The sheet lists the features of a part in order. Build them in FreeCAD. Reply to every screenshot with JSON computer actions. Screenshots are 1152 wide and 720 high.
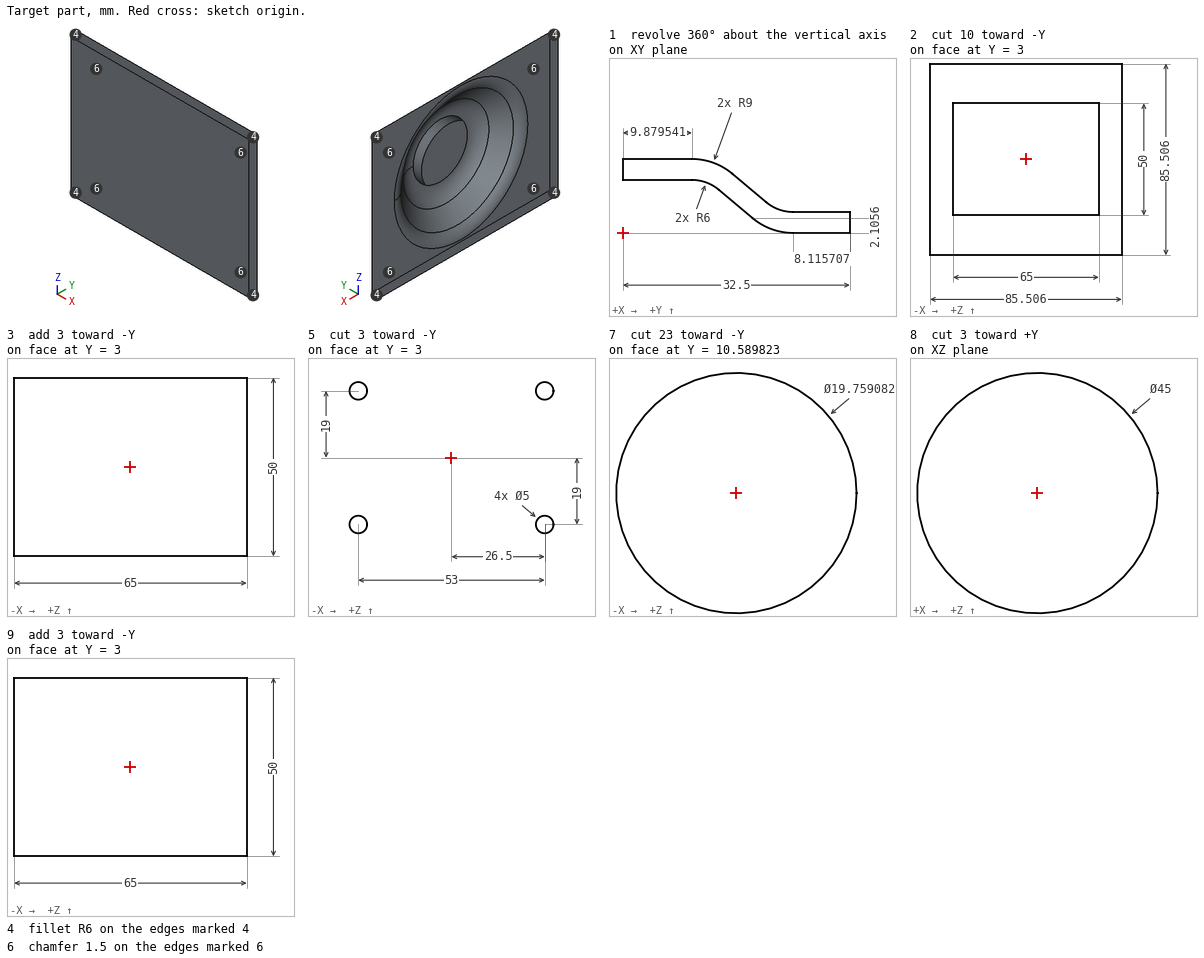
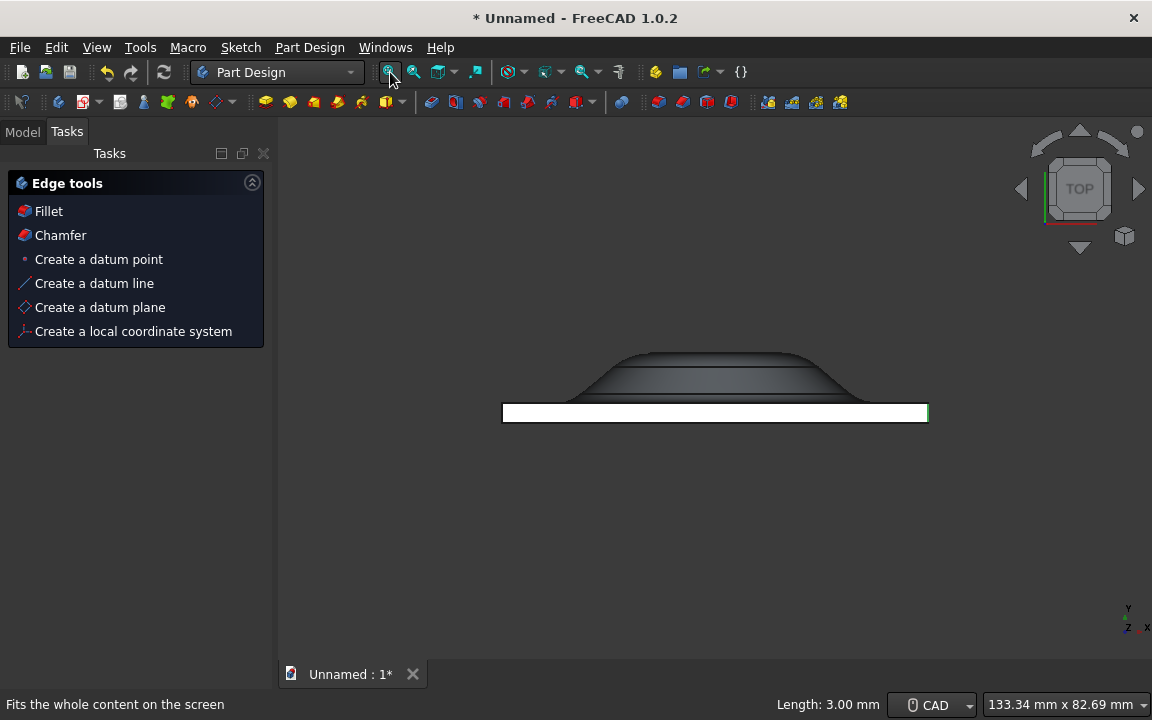
{"action": "left_click", "coordinate": [502, 412], "text": "ctrl"}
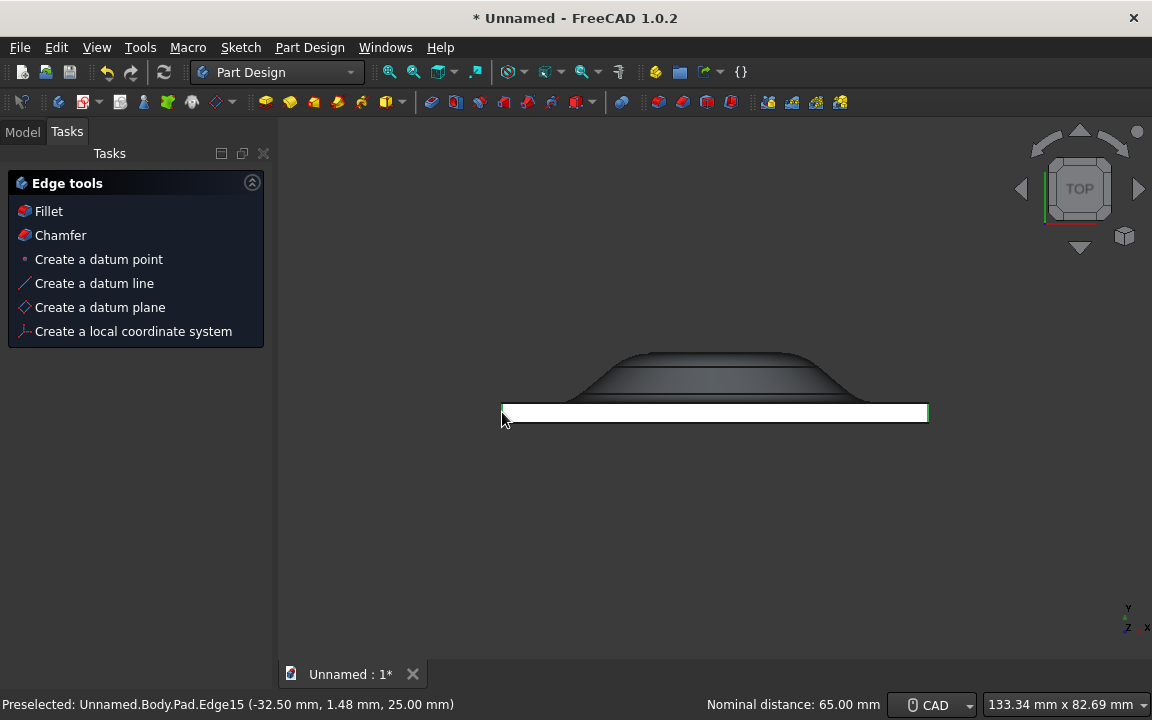
{"action": "scroll", "coordinate": [928, 412], "scroll_direction": "up", "scroll_amount": 4}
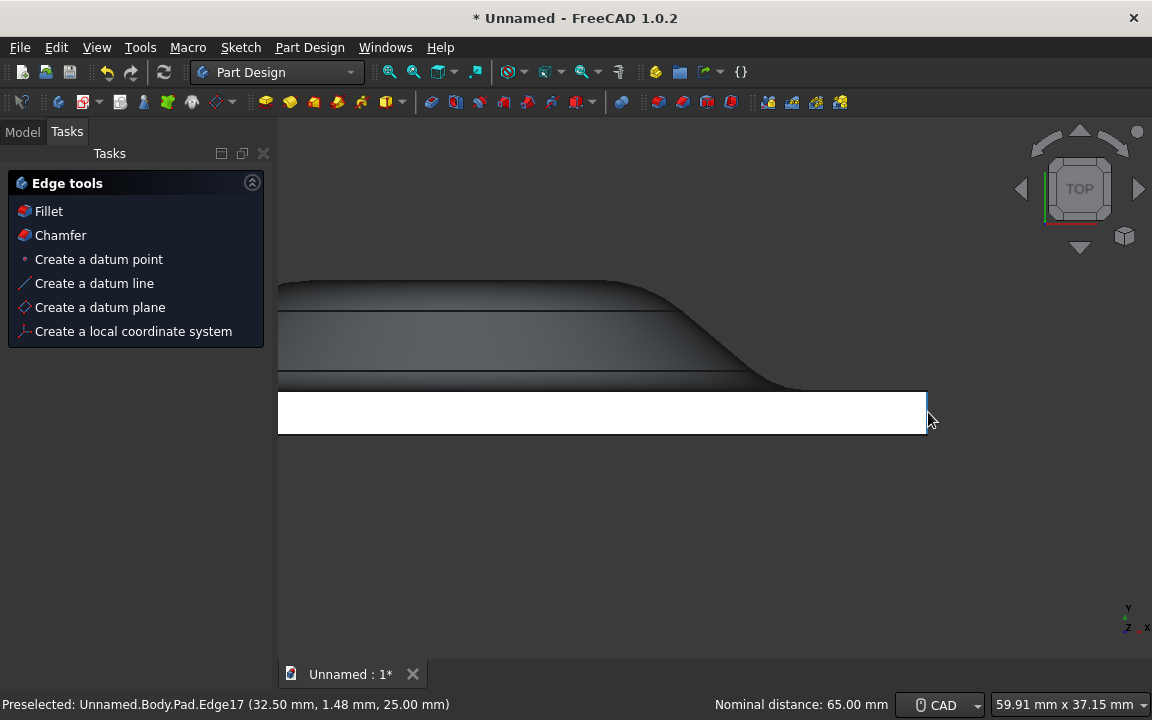
{"action": "left_click", "coordinate": [390, 72]}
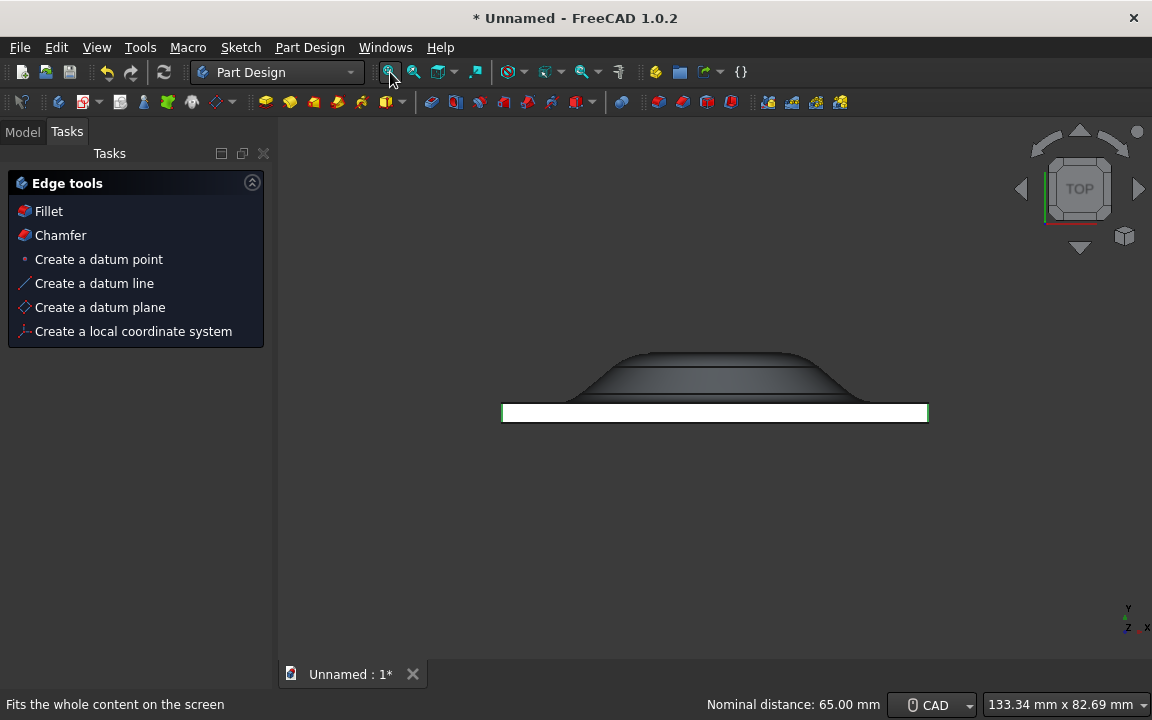
{"action": "key", "text": "1"}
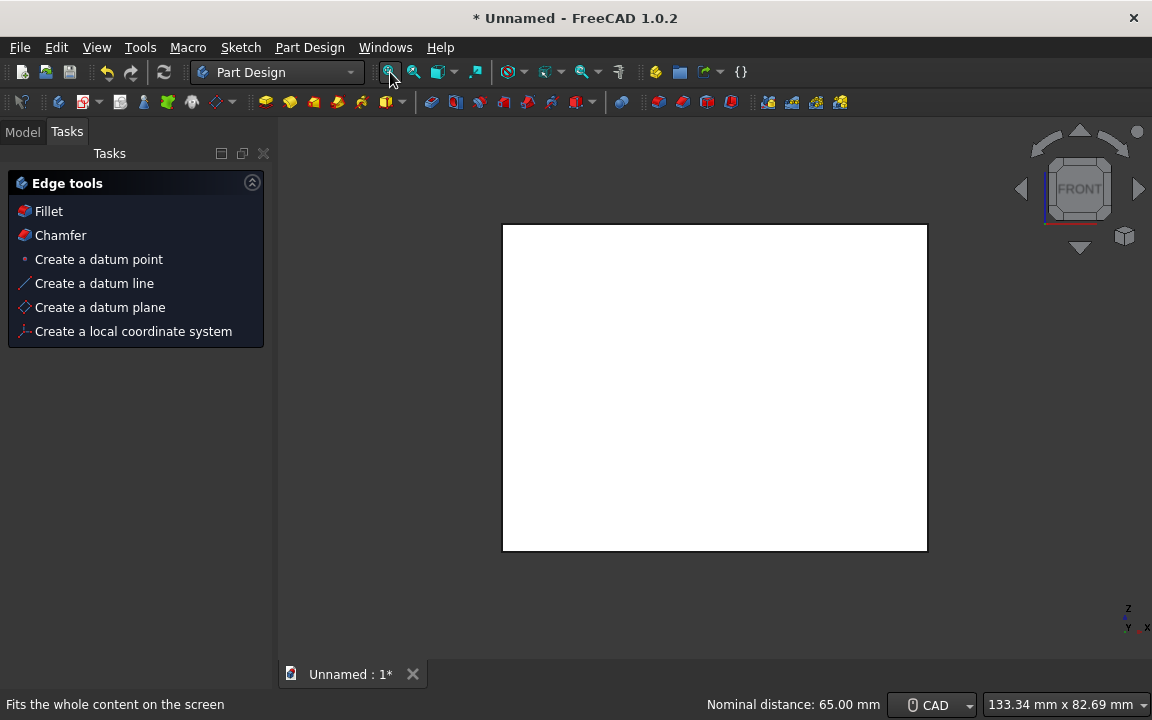
{"action": "scroll", "coordinate": [928, 551], "scroll_direction": "up", "scroll_amount": 4}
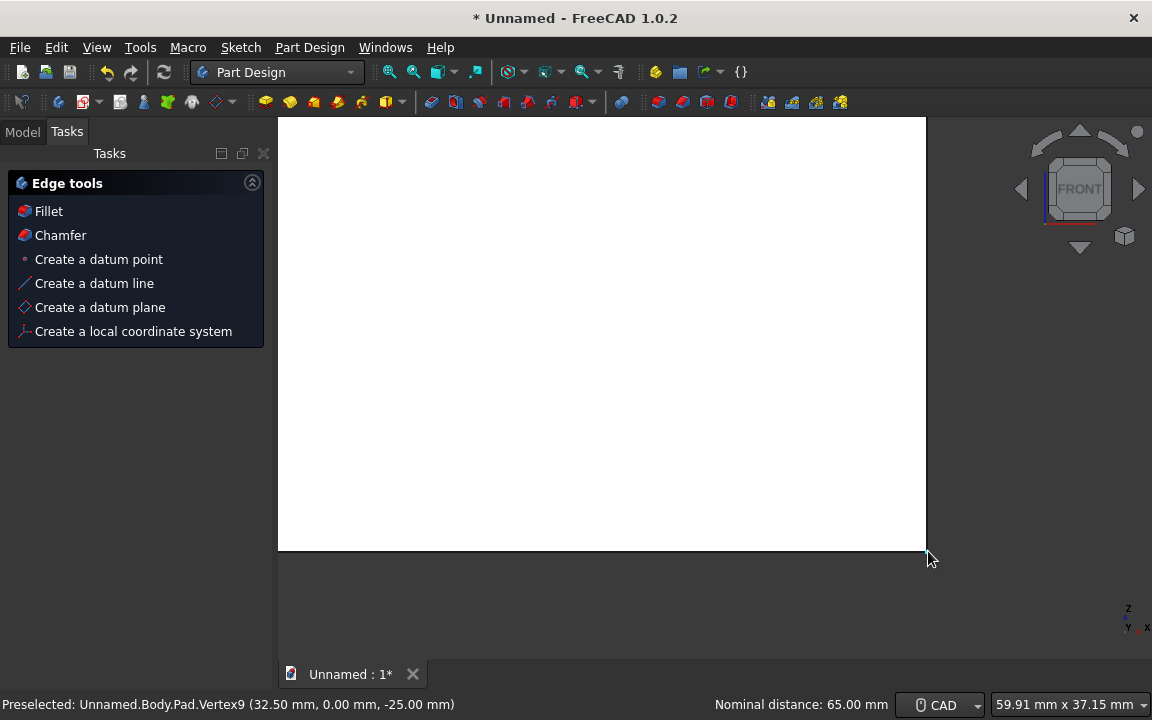
{"action": "left_click", "coordinate": [390, 72]}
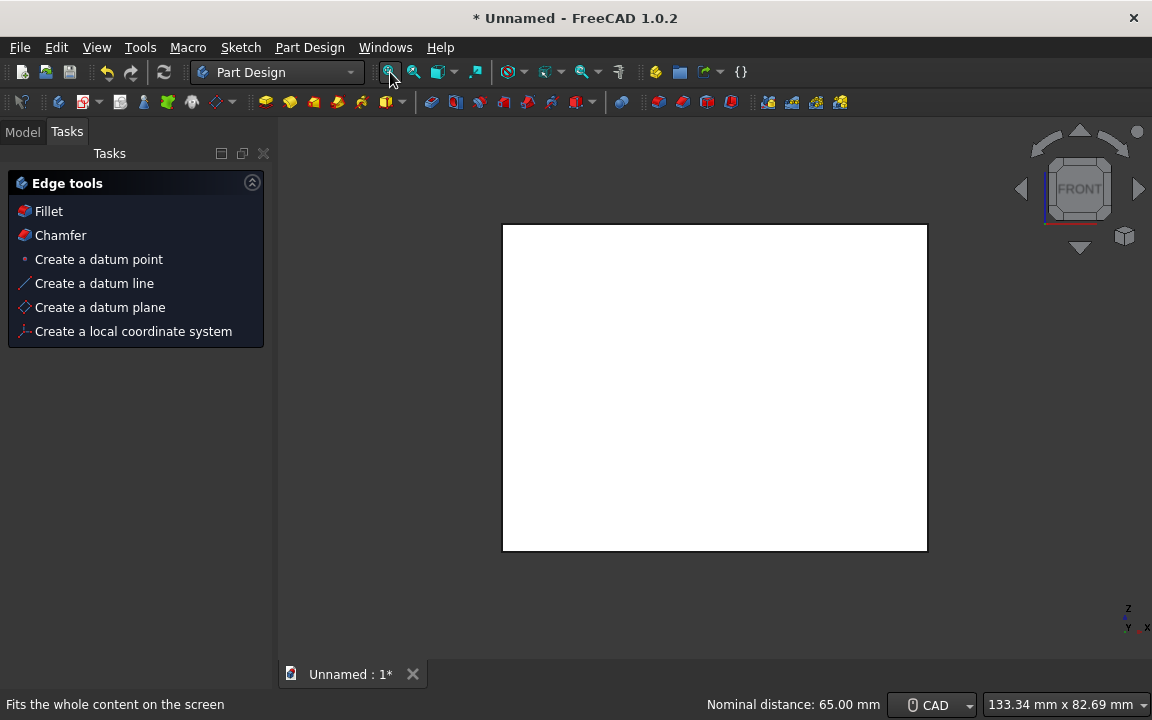
{"action": "key", "text": "3"}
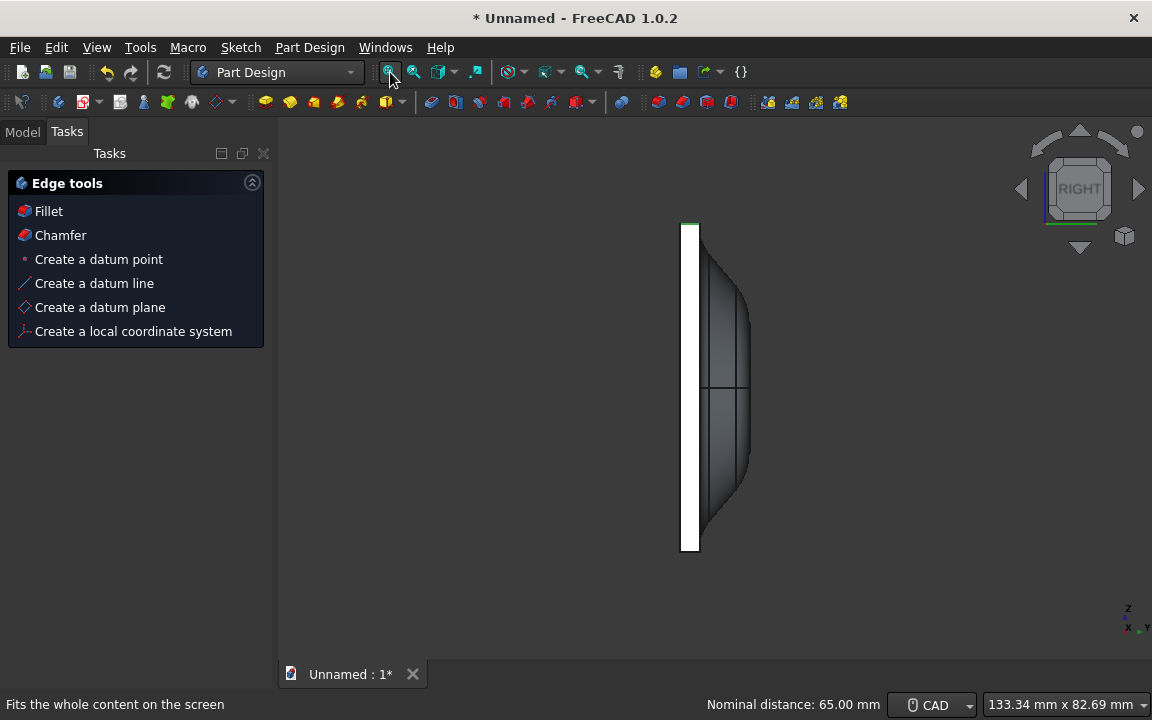
{"action": "left_click", "coordinate": [690, 551], "text": "ctrl"}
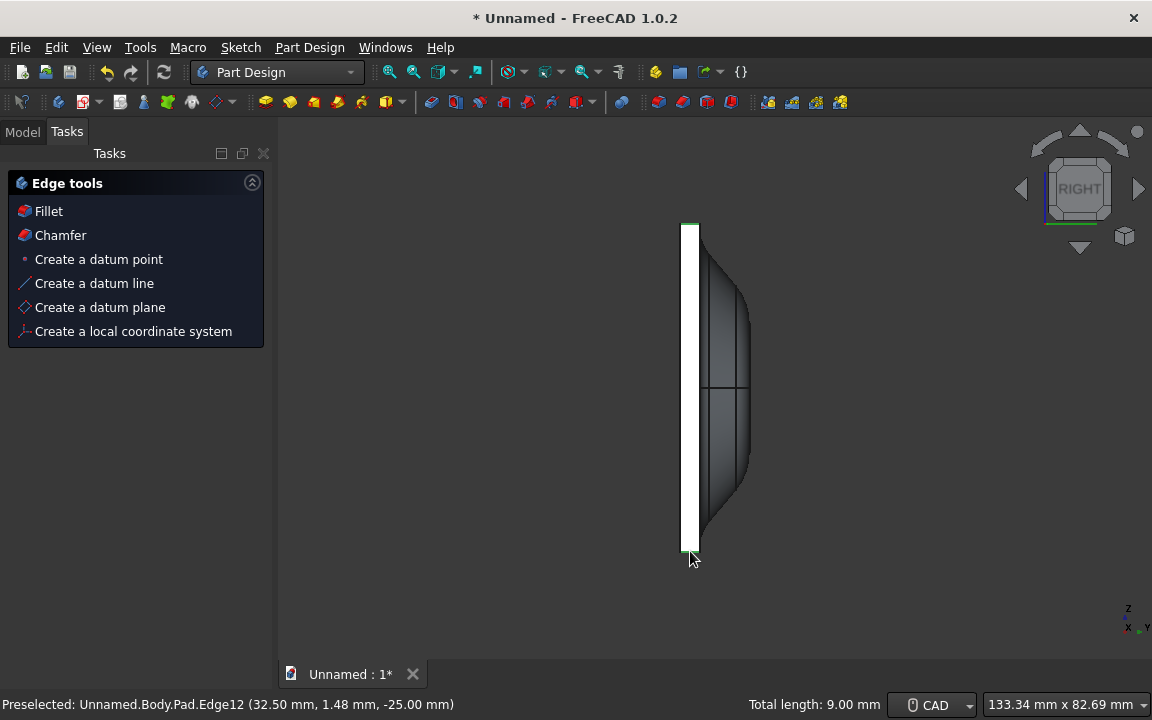
{"action": "scroll", "coordinate": [690, 551], "scroll_direction": "up", "scroll_amount": 4}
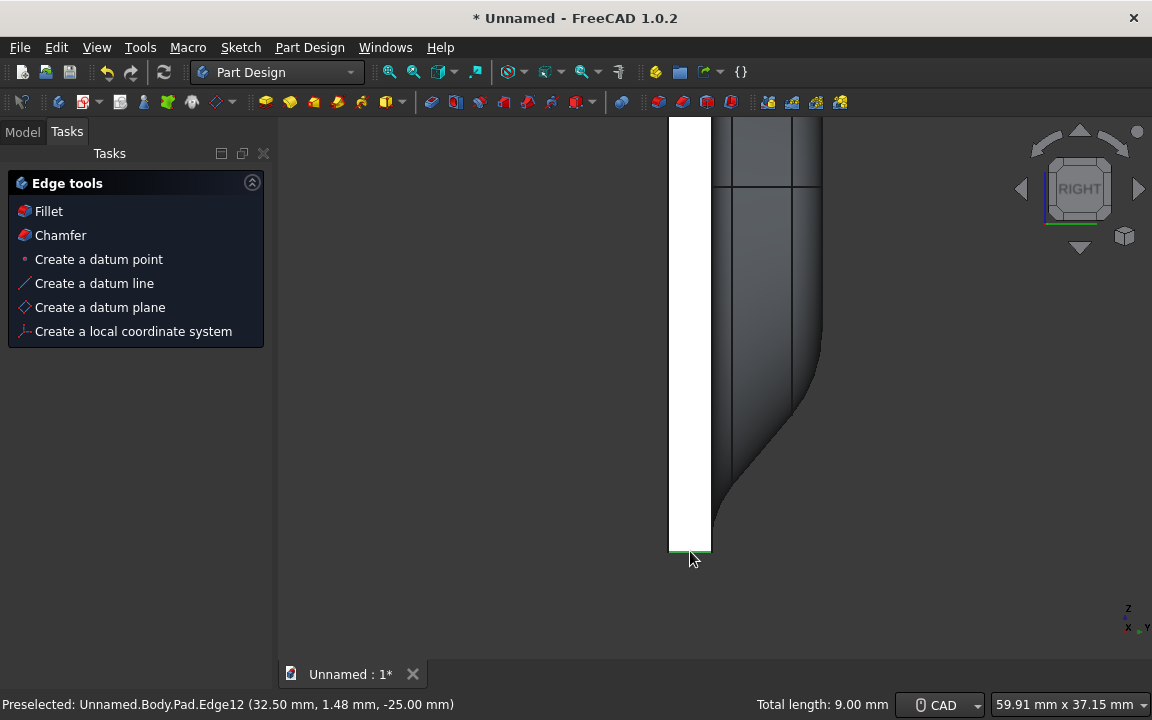
{"action": "left_click", "coordinate": [390, 72]}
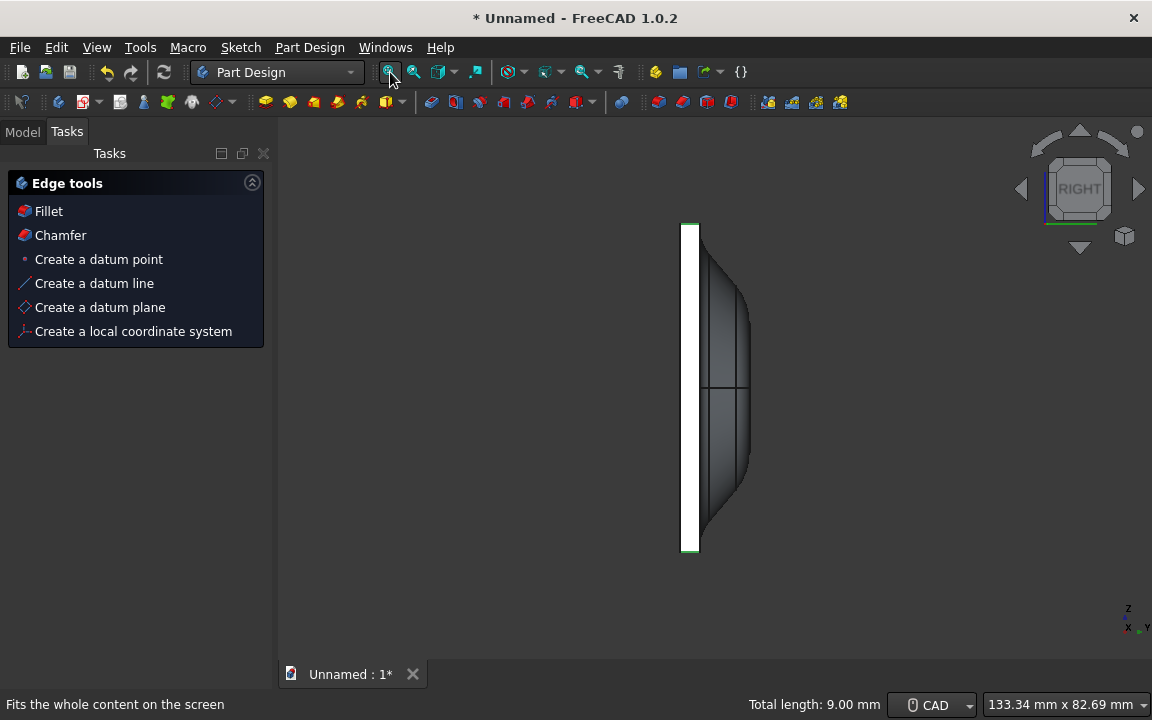
{"action": "key", "text": "5"}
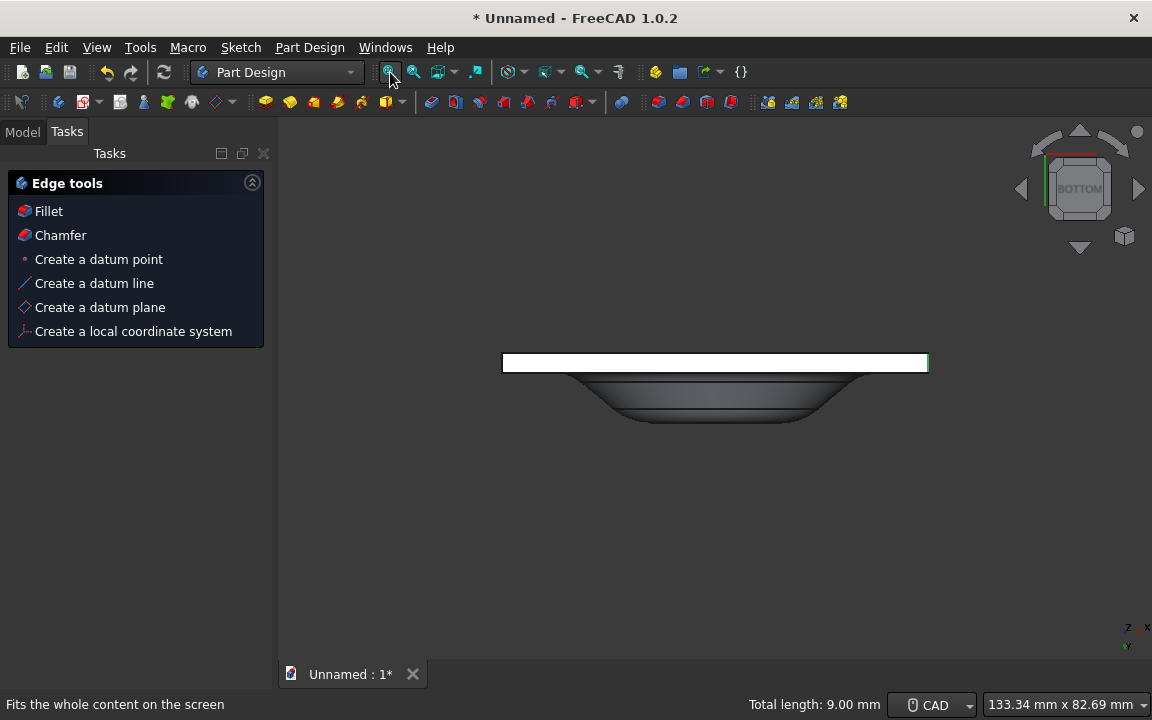
{"action": "left_click", "coordinate": [502, 362], "text": "ctrl"}